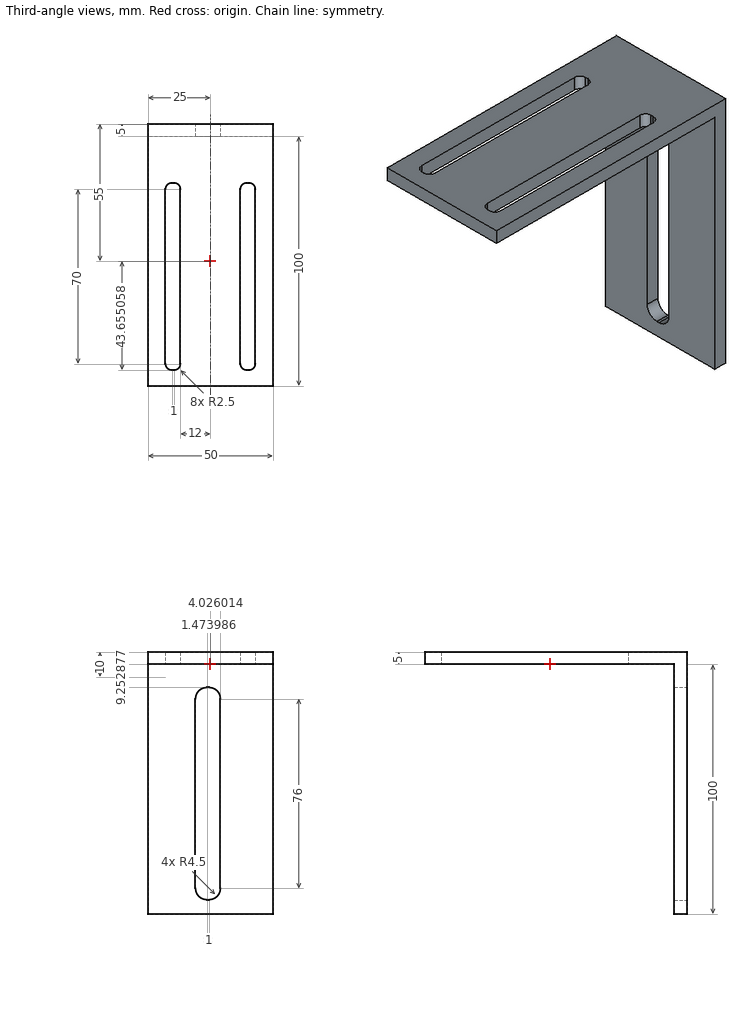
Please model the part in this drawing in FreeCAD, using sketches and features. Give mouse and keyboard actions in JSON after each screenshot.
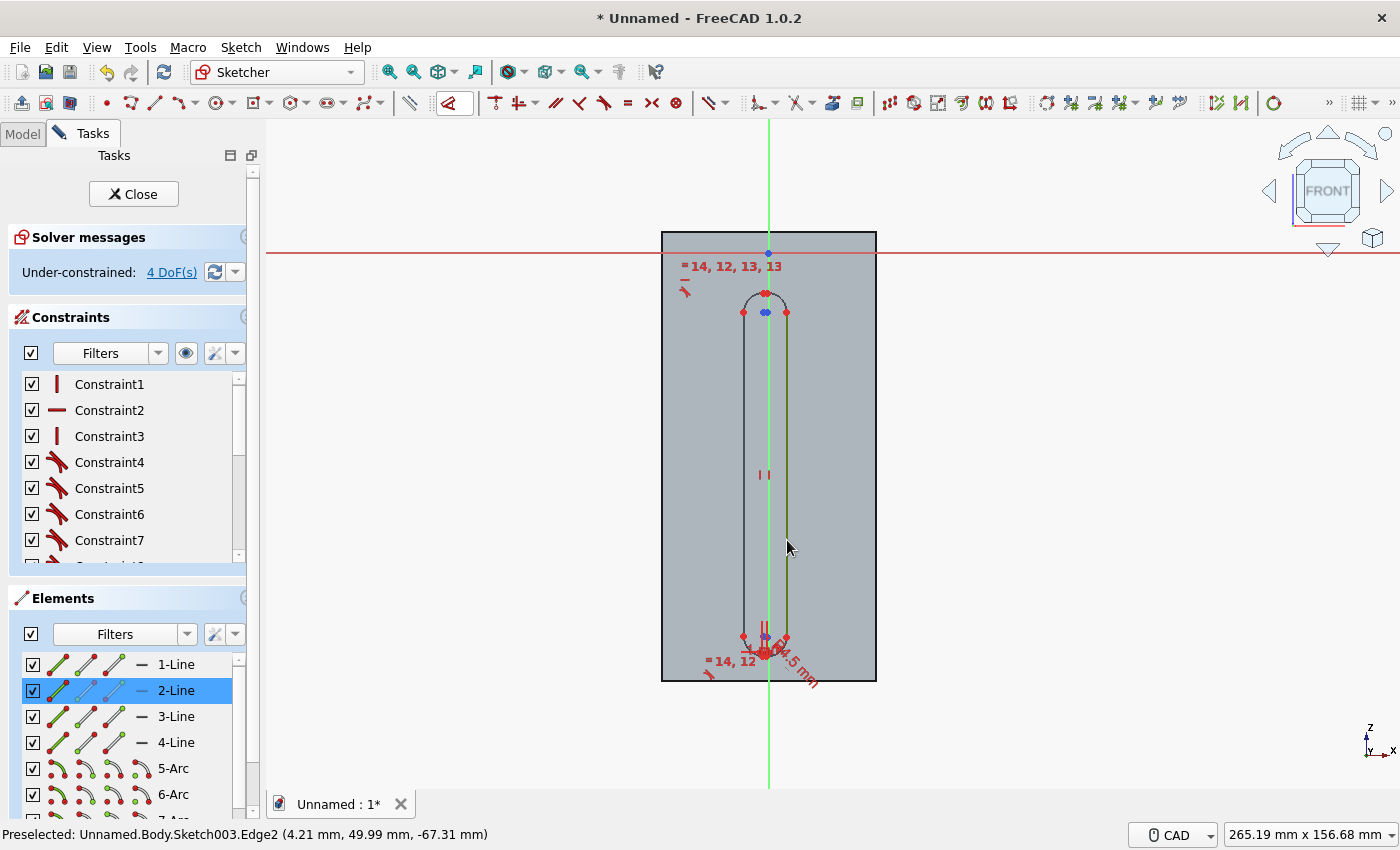
{"action": "left_click", "coordinate": [468, 104]}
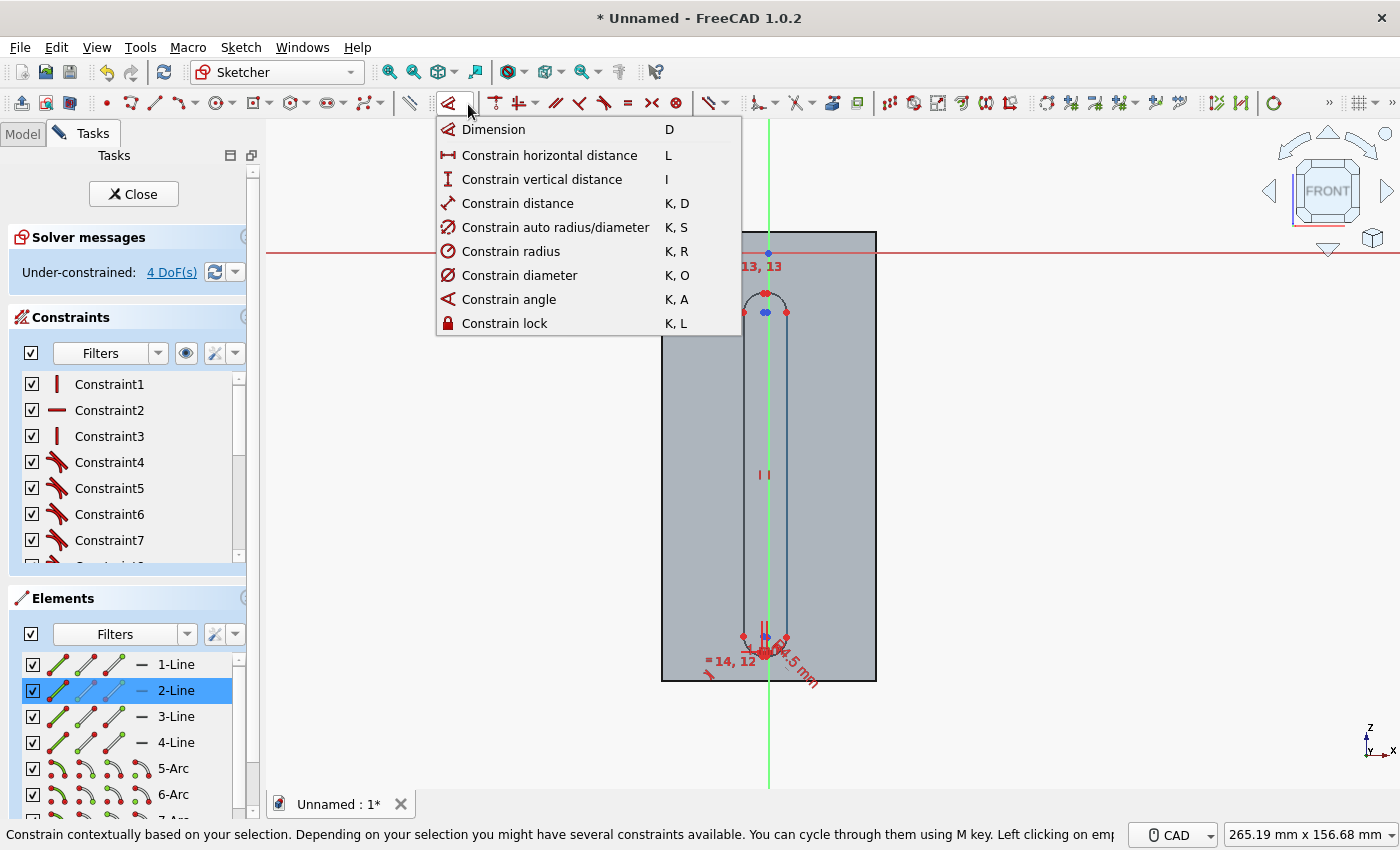
{"action": "left_click", "coordinate": [589, 179]}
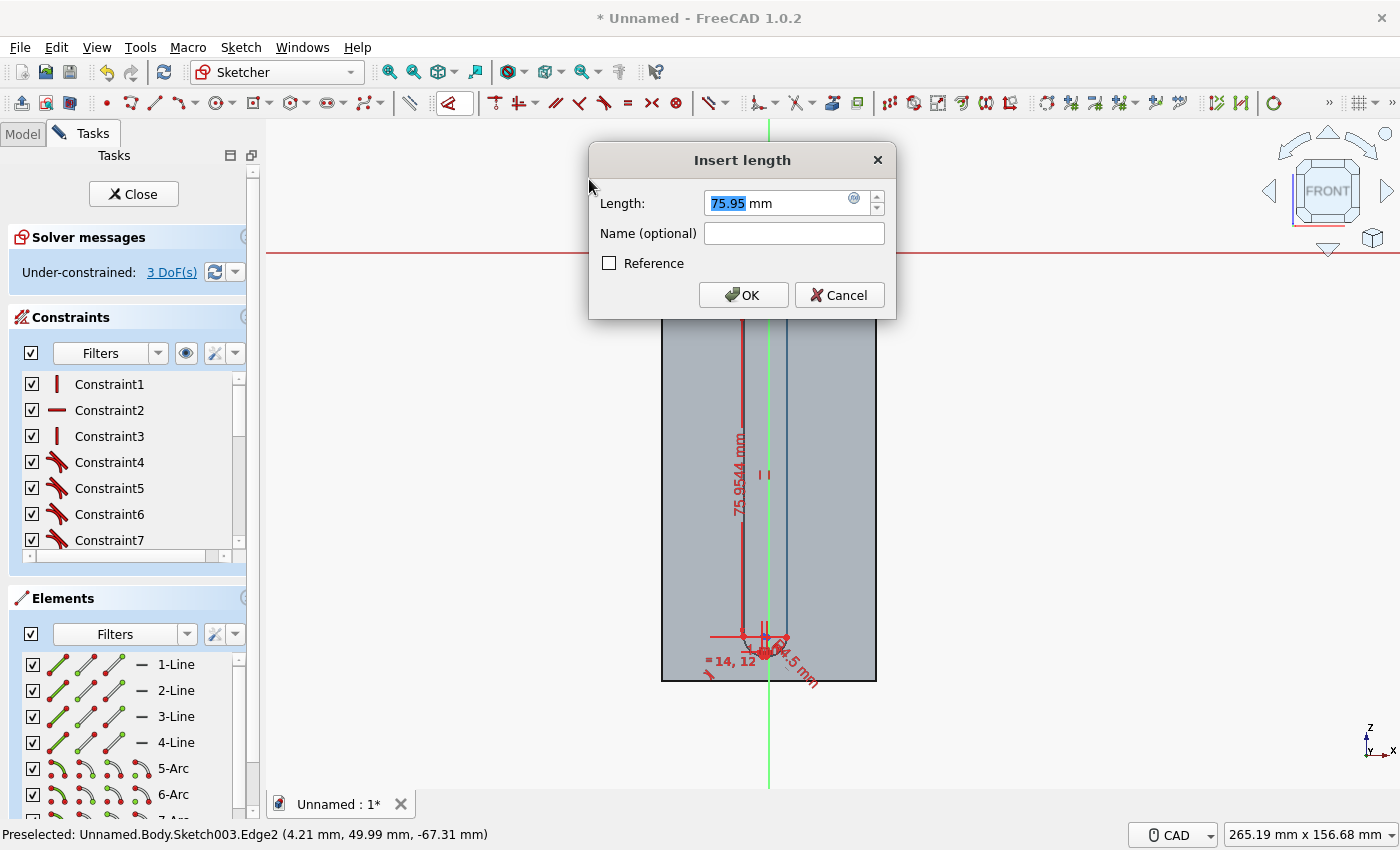
{"action": "type", "text": "76"}
{"action": "key", "text": "Return"}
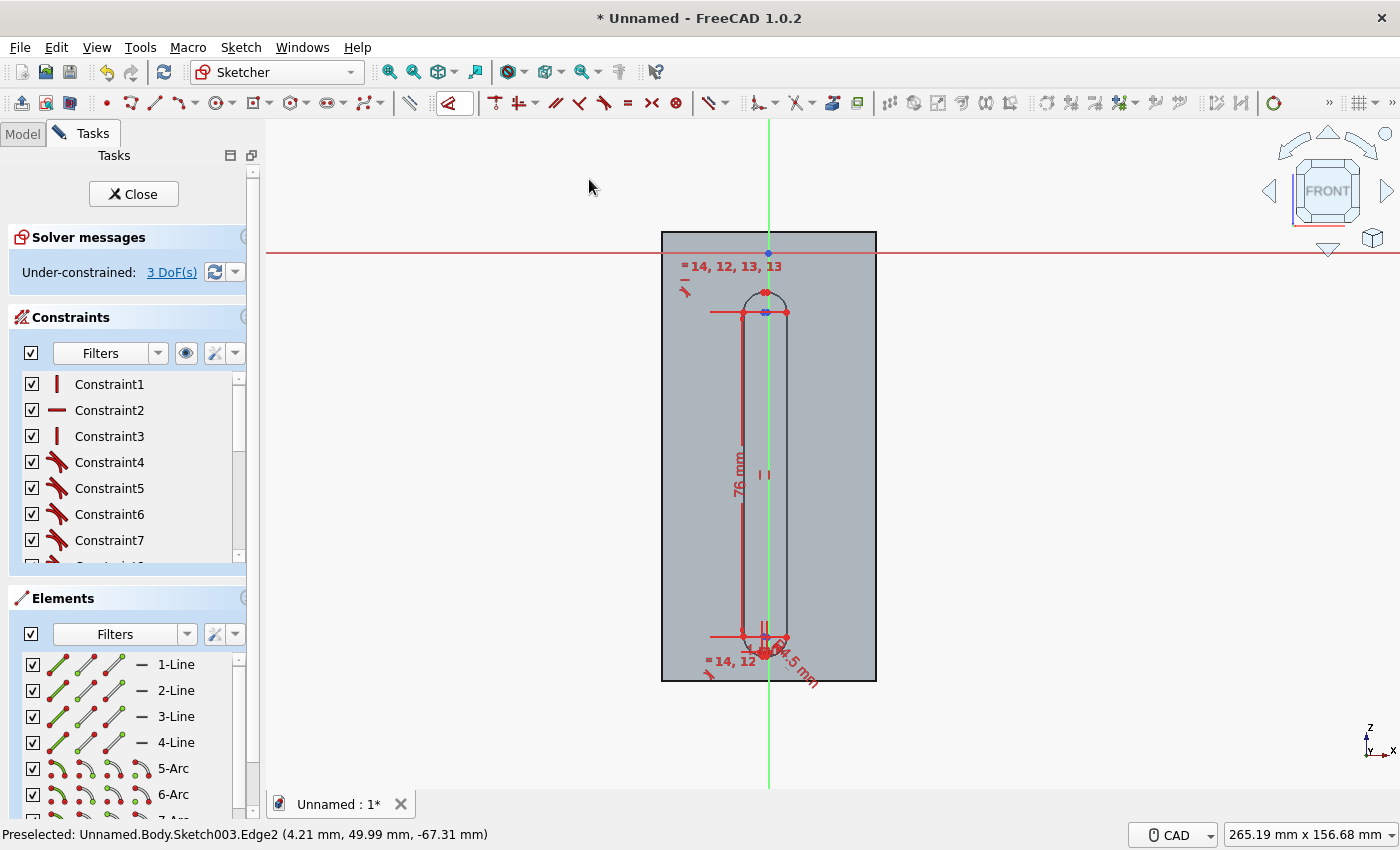
{"action": "scroll", "coordinate": [762, 656], "scroll_direction": "up", "scroll_amount": 10}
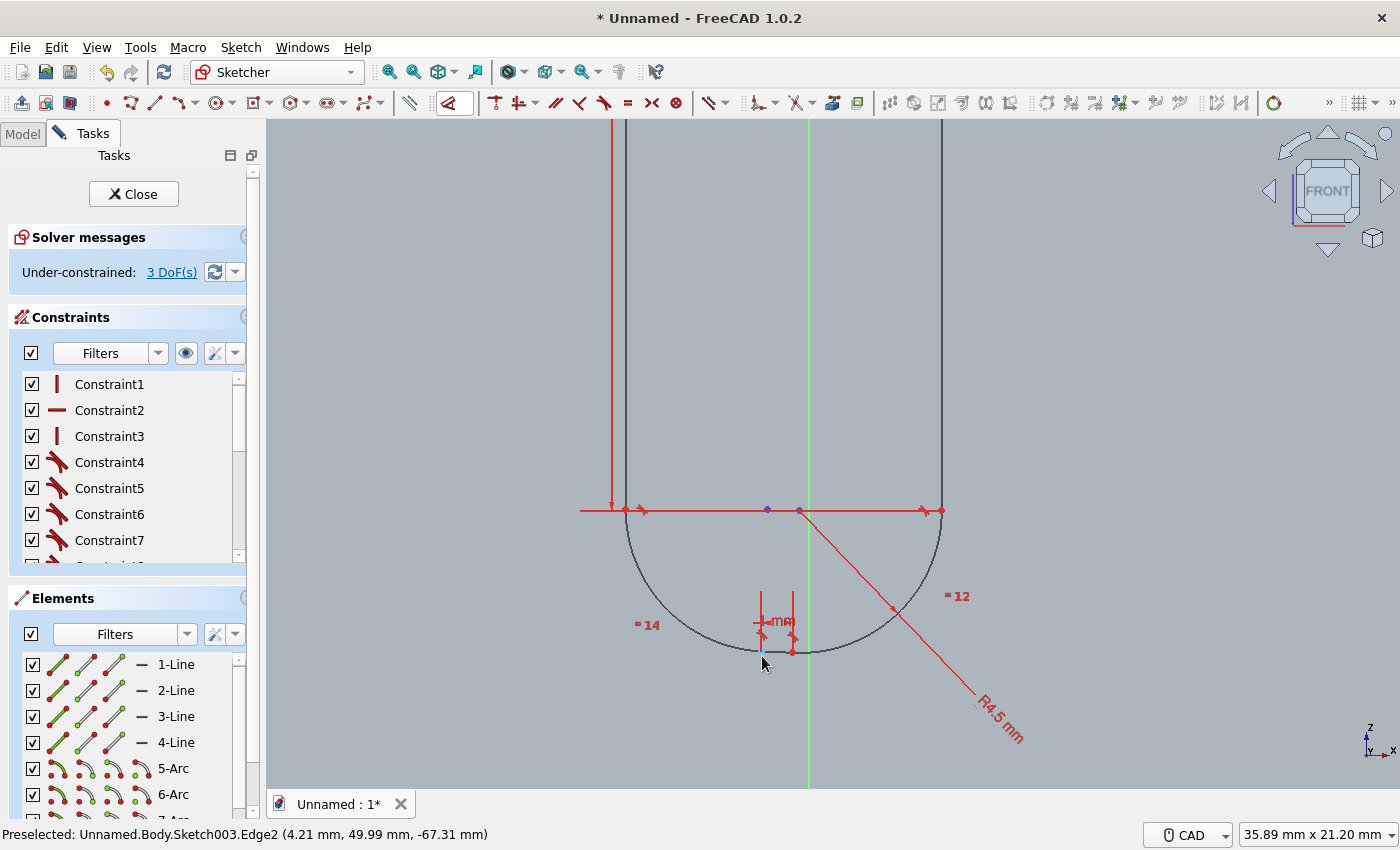
{"action": "left_click", "coordinate": [761, 651]}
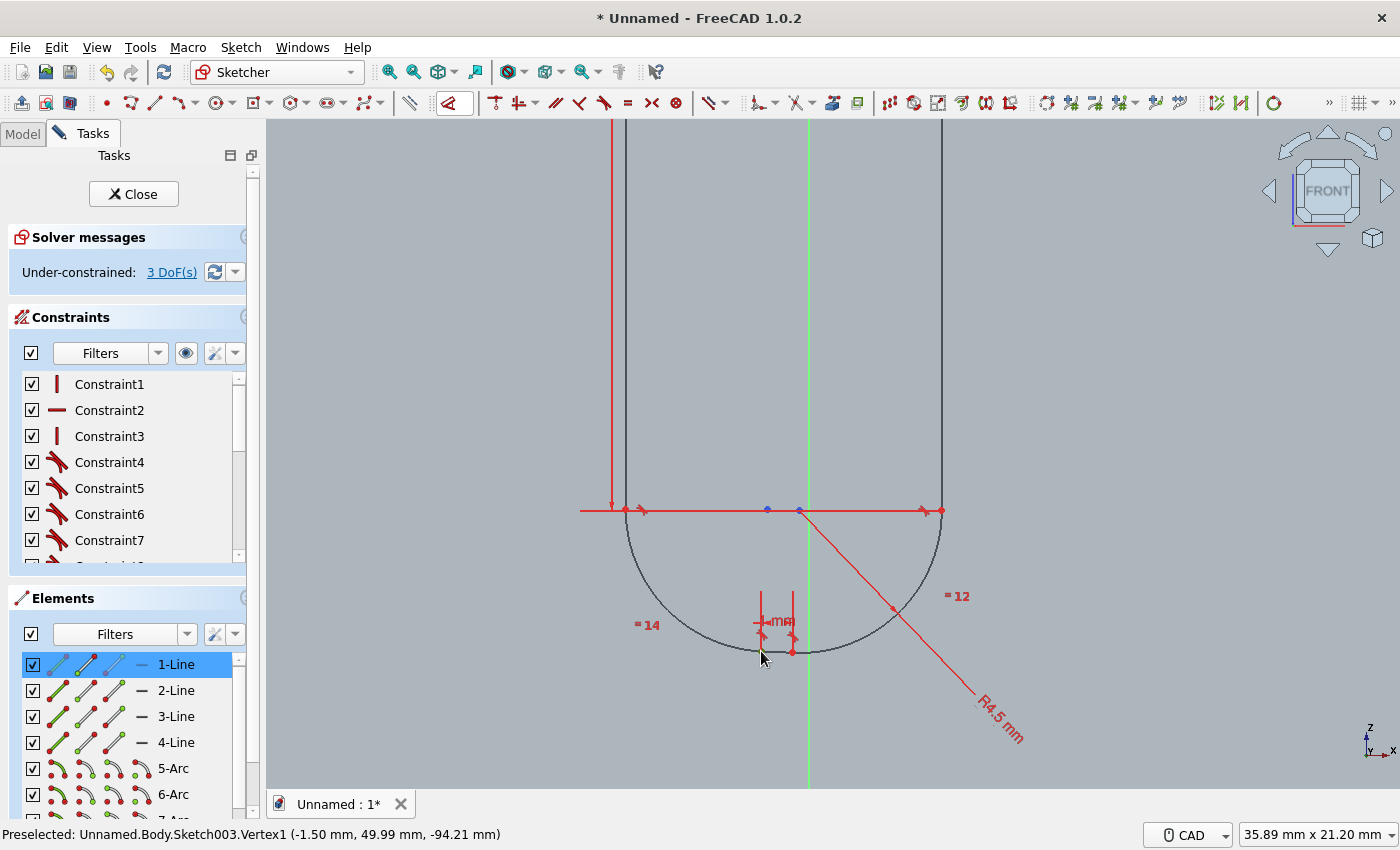
{"action": "key", "text": "l"}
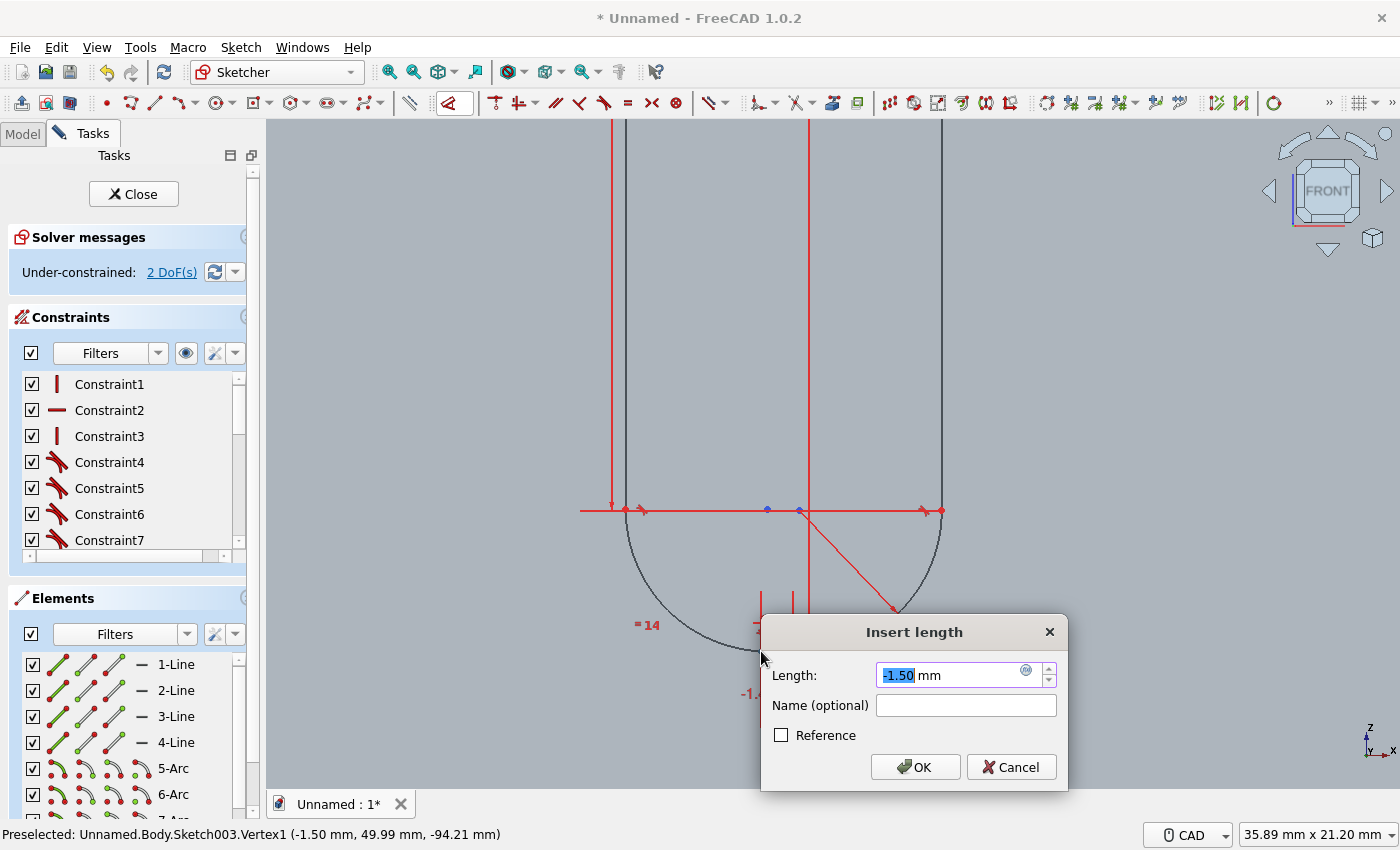
{"action": "type", "text": "-1.473986"}
{"action": "key", "text": "Return"}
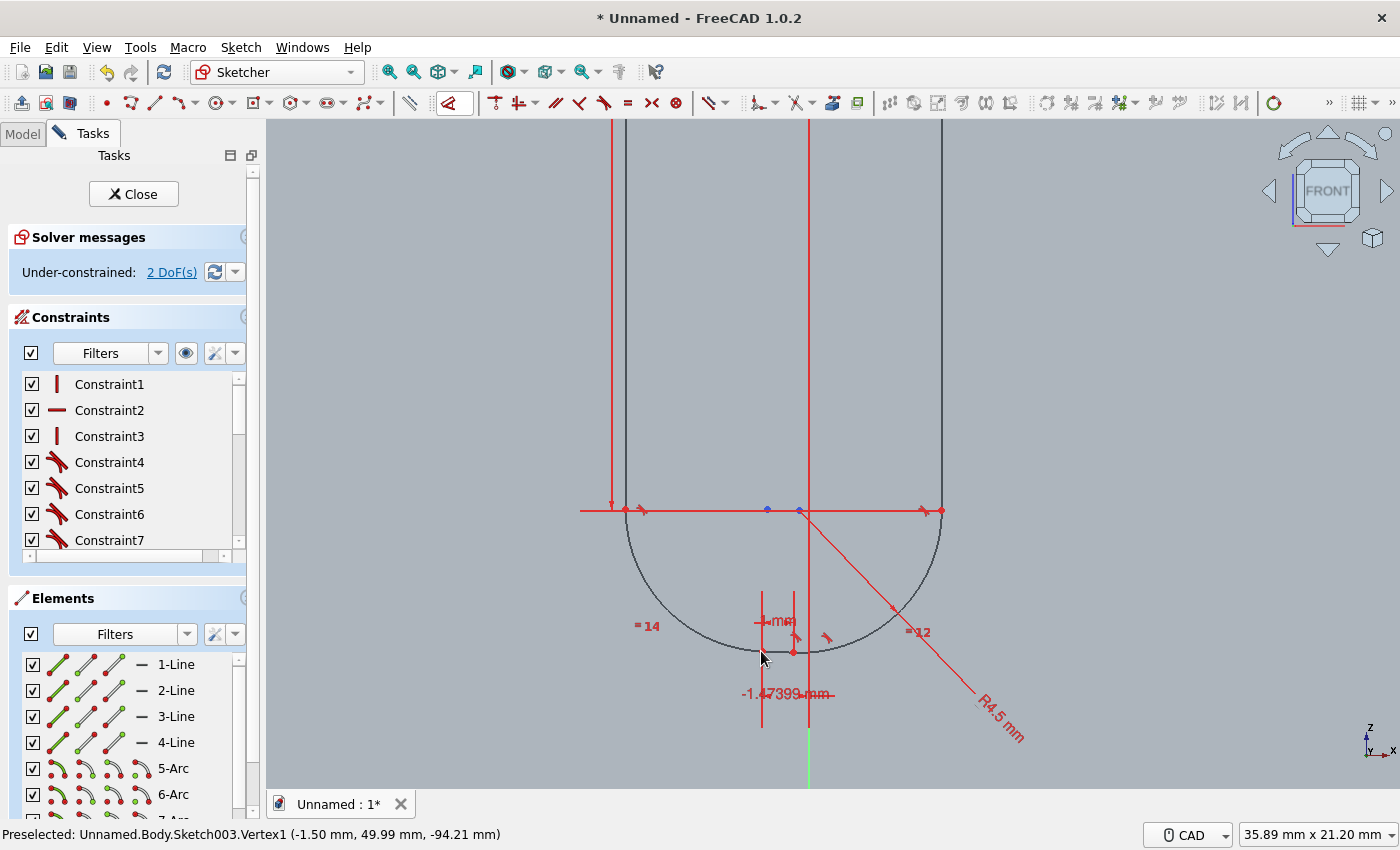
{"action": "scroll", "coordinate": [762, 656], "scroll_direction": "down", "scroll_amount": 10}